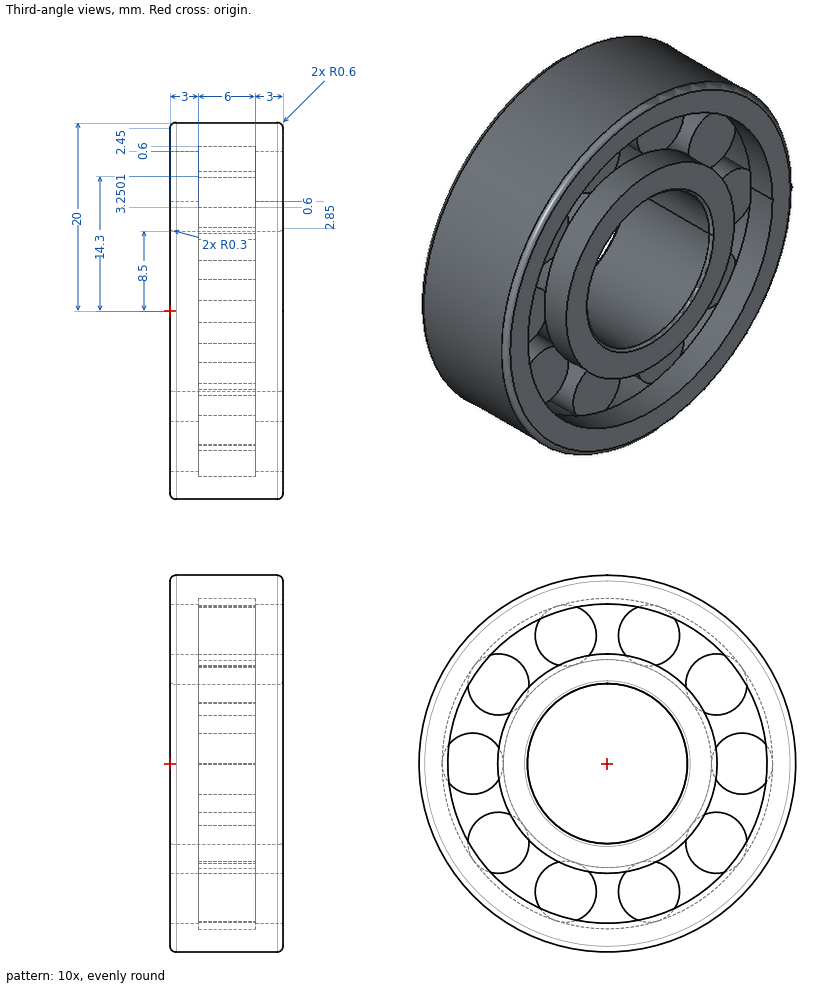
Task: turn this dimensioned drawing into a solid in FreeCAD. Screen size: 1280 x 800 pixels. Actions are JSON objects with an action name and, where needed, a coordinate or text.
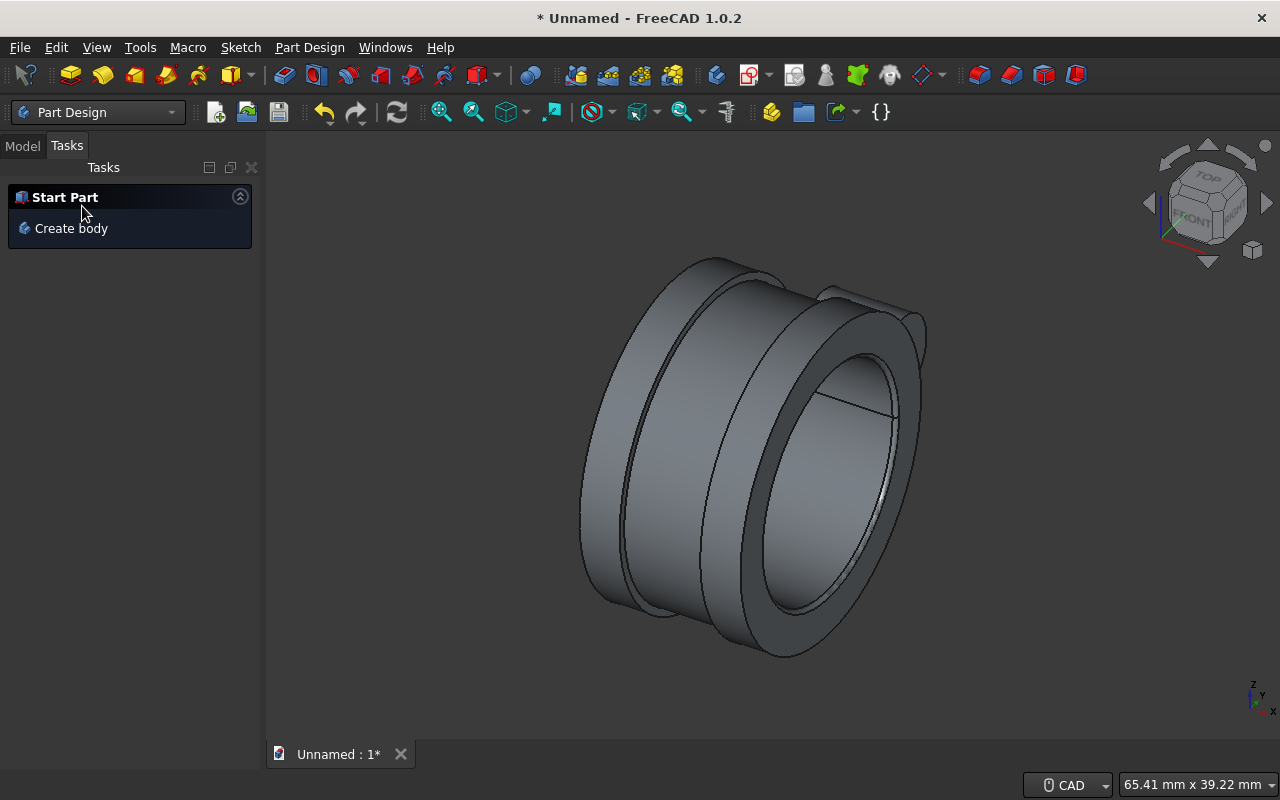
{"action": "left_click", "coordinate": [750, 76]}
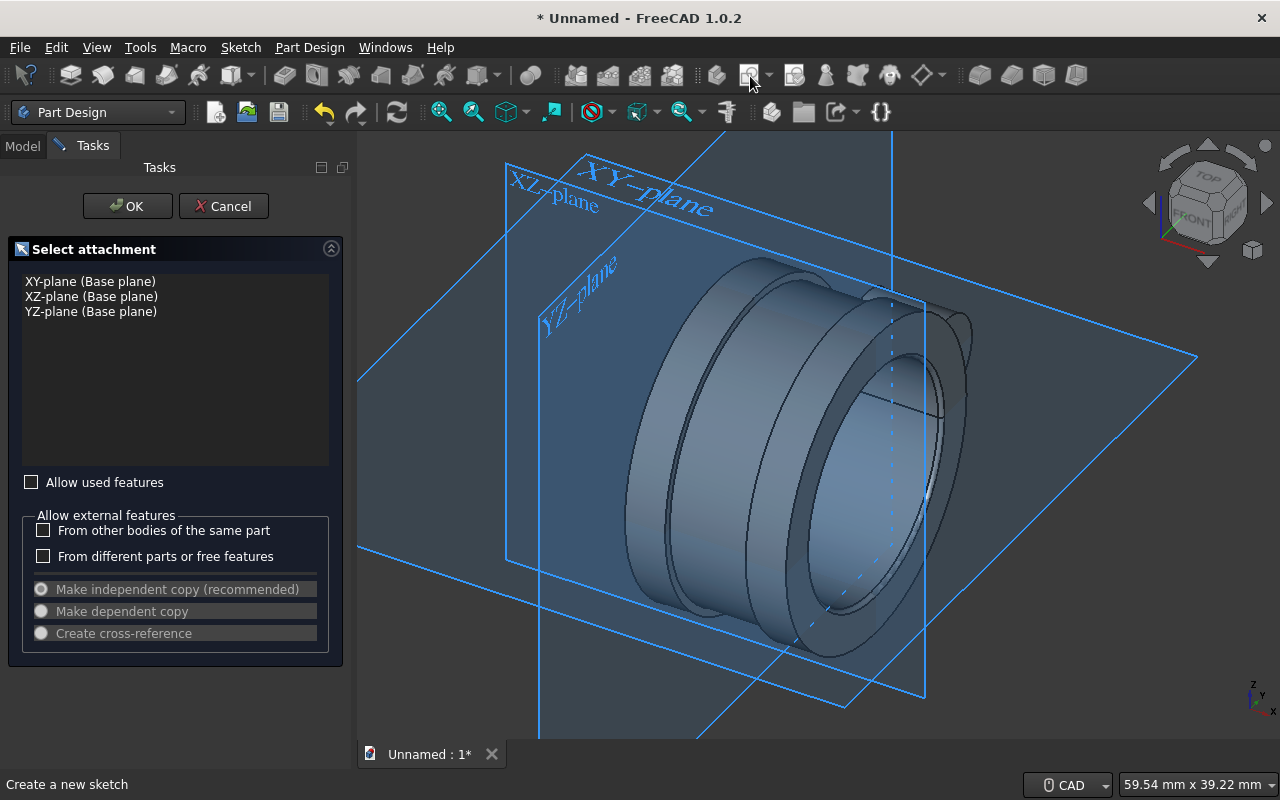
{"action": "left_click", "coordinate": [82, 282]}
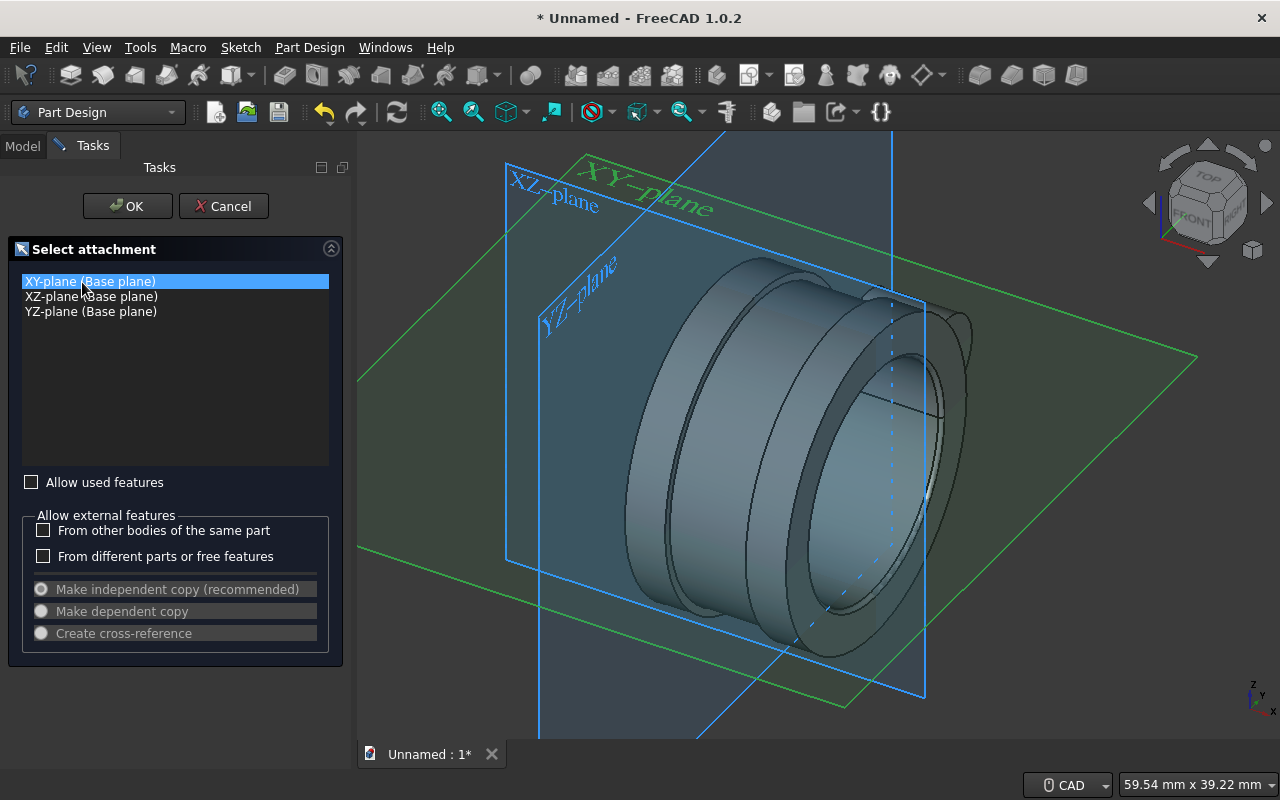
{"action": "left_click", "coordinate": [128, 206]}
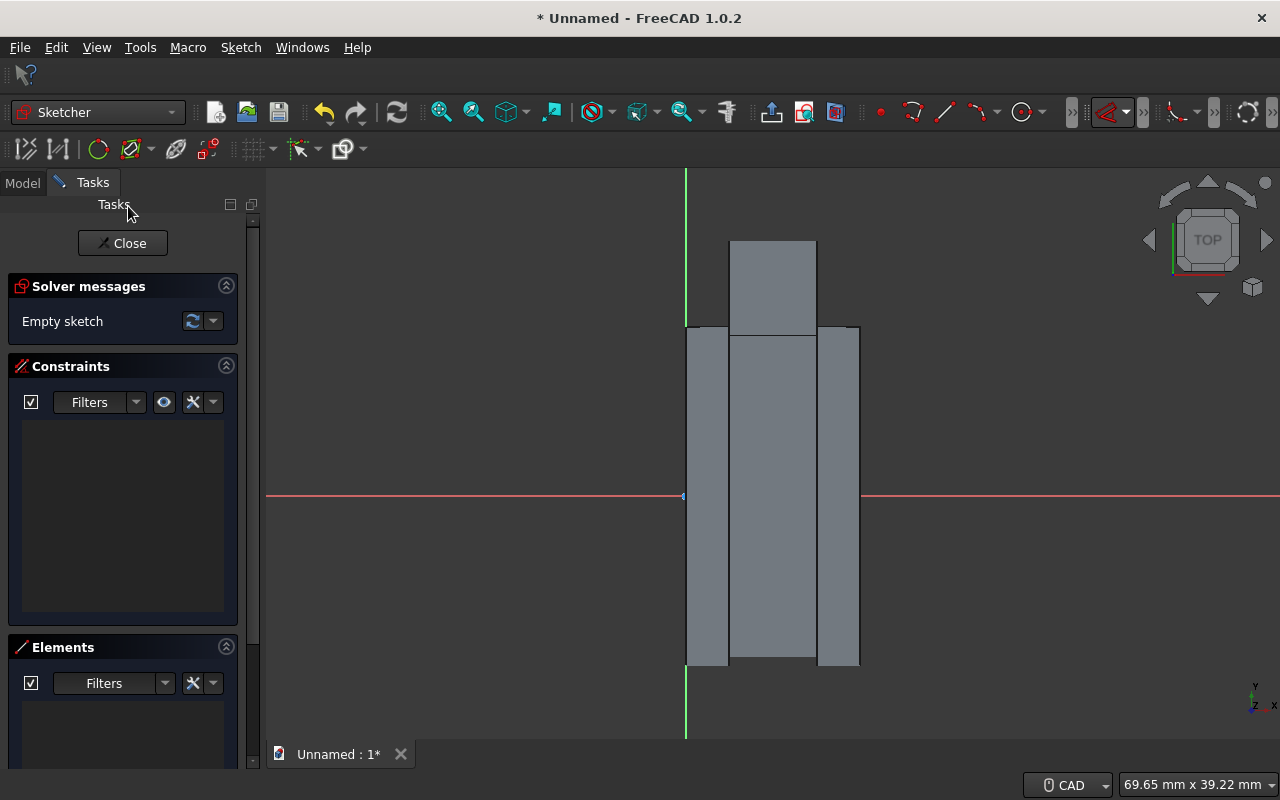
{"action": "left_click", "coordinate": [836, 112]}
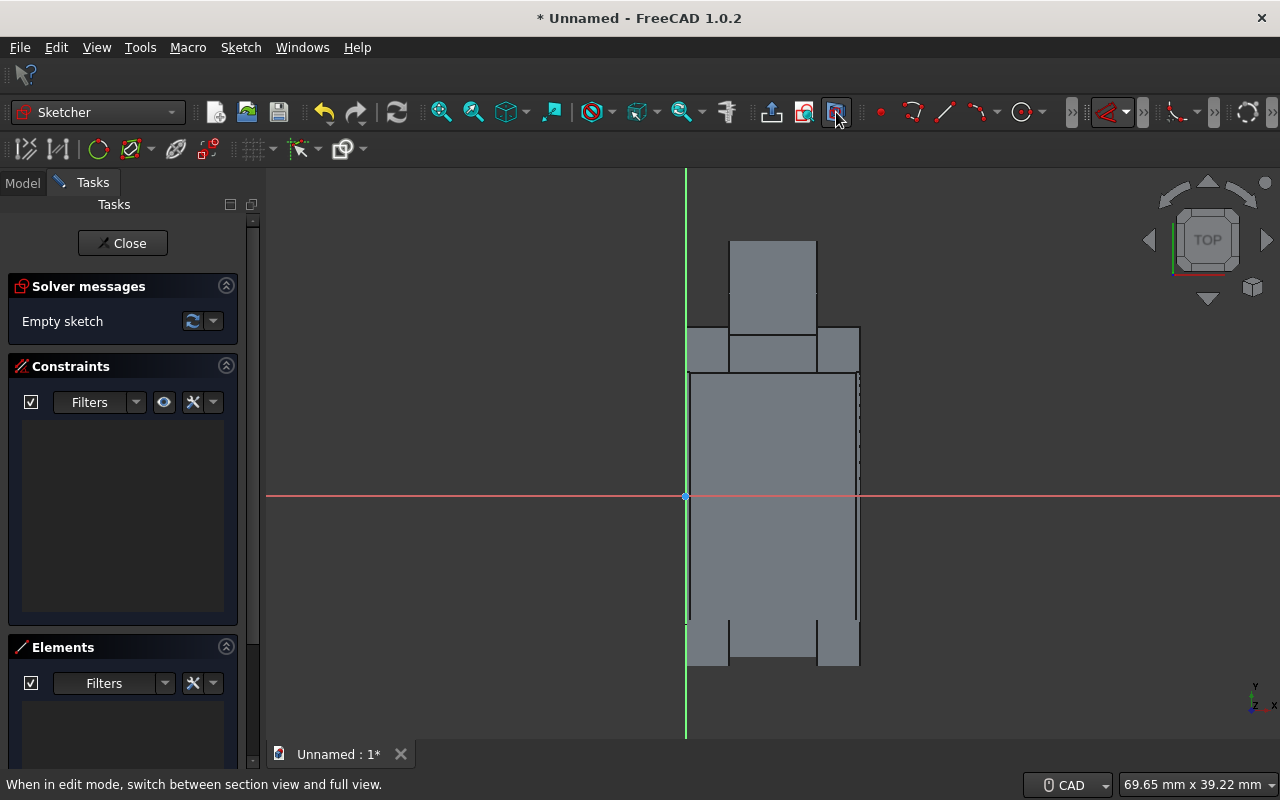
{"action": "scroll", "coordinate": [395, 711], "scroll_direction": "down", "scroll_amount": 1}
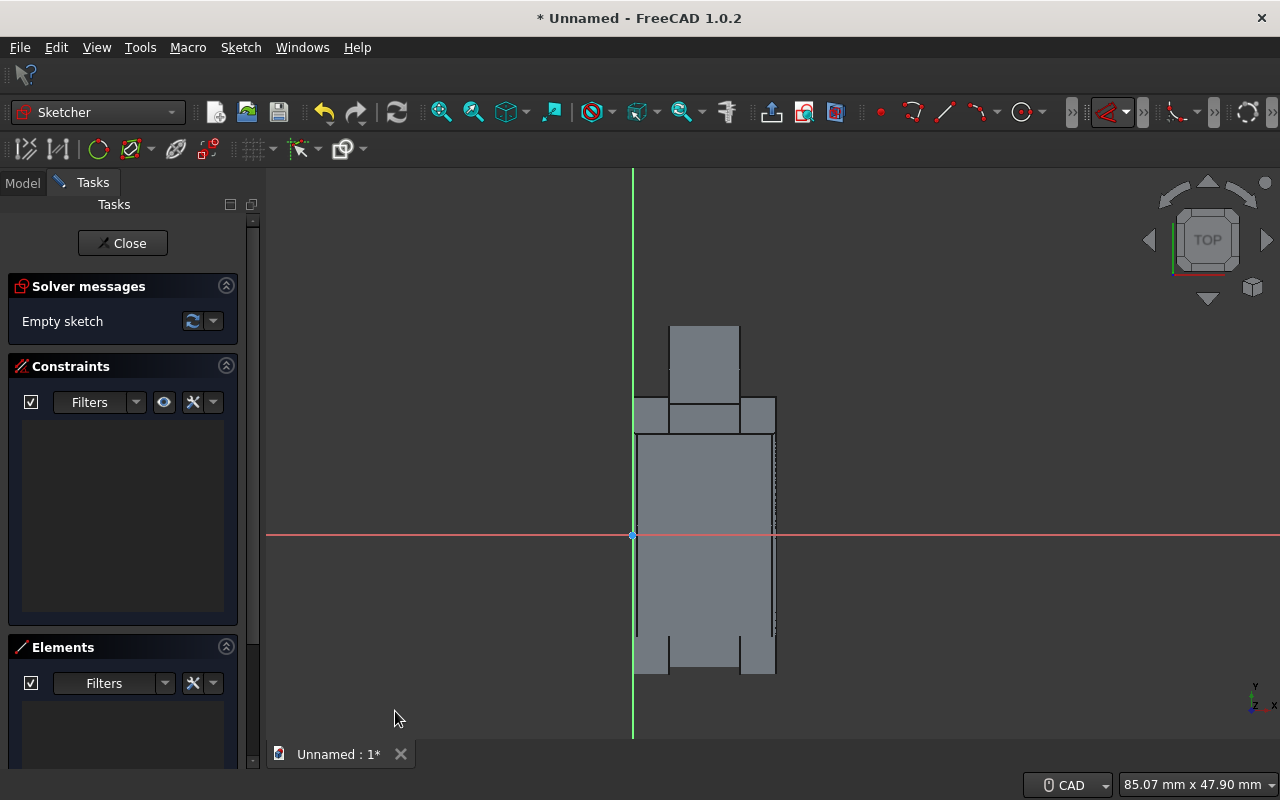
{"action": "scroll", "coordinate": [705, 340], "scroll_direction": "up", "scroll_amount": 2}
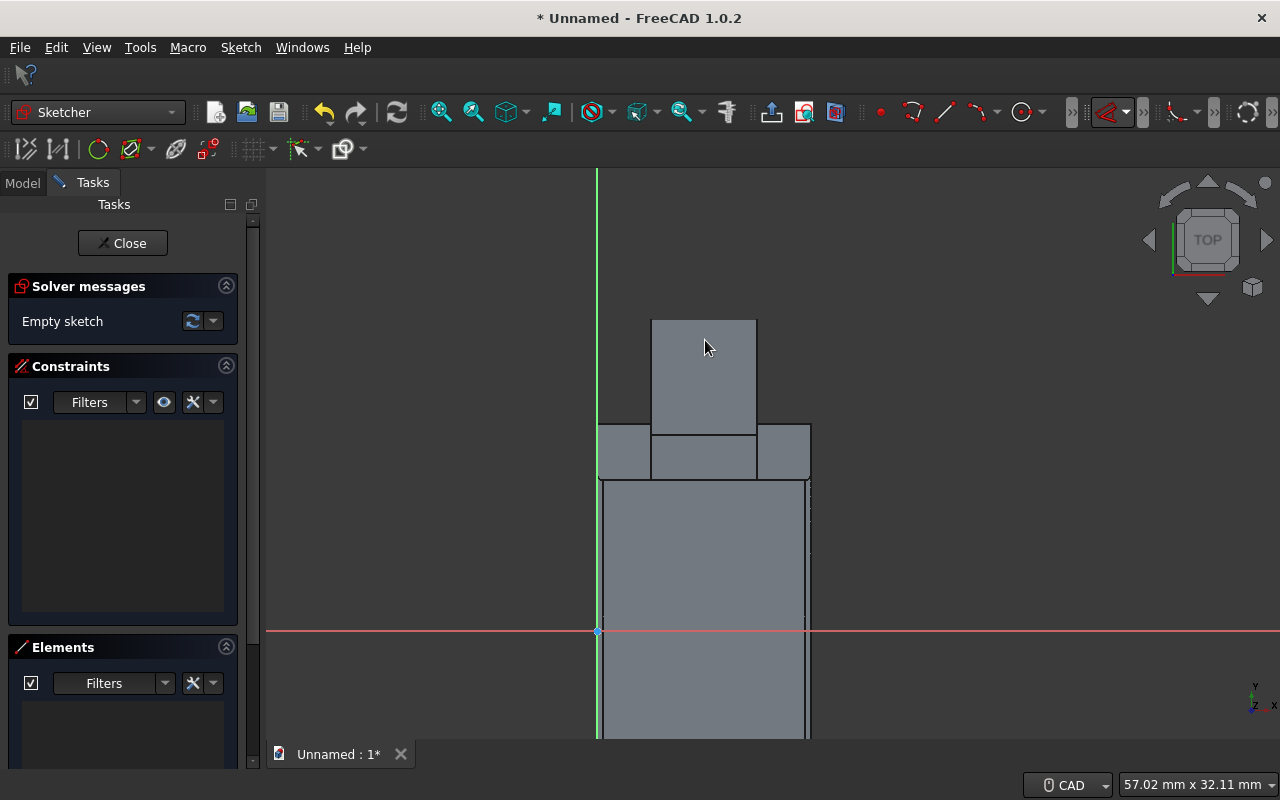
{"action": "left_click", "coordinate": [946, 112]}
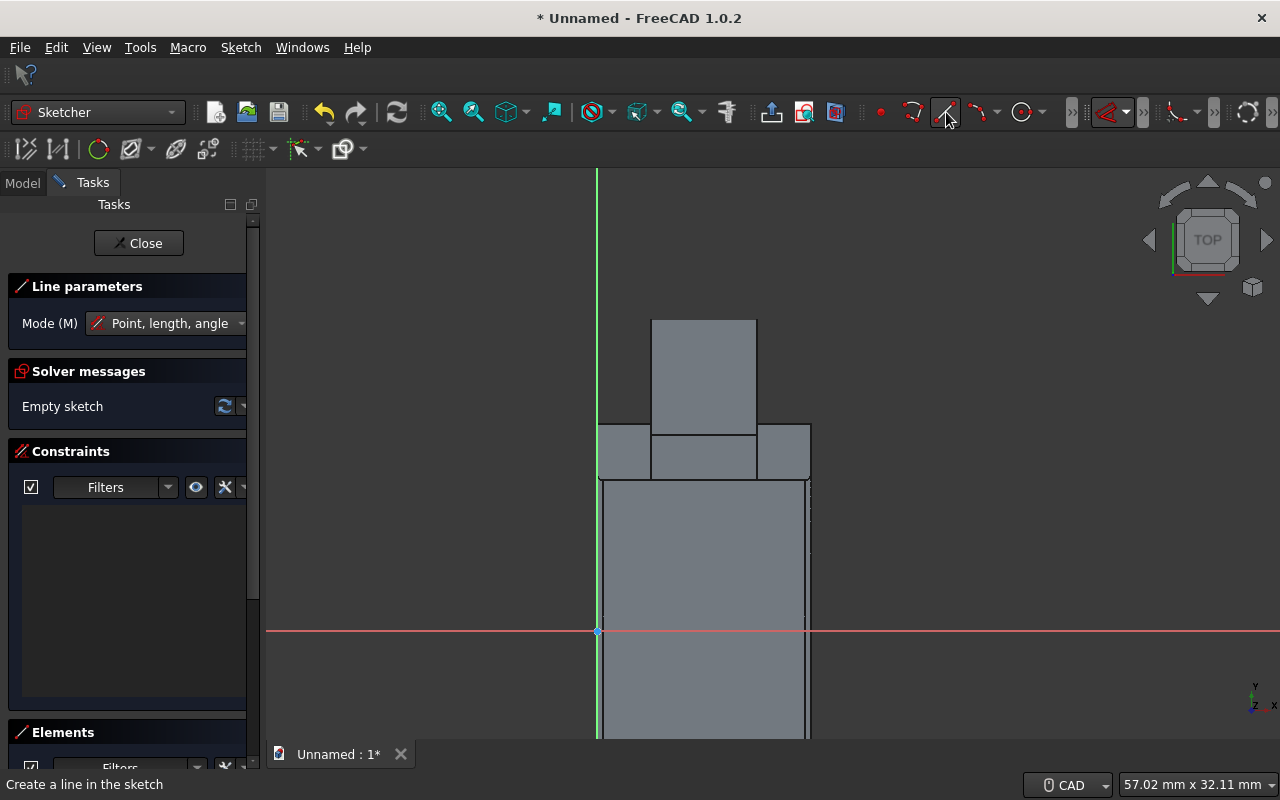
{"action": "left_click", "coordinate": [800, 276]}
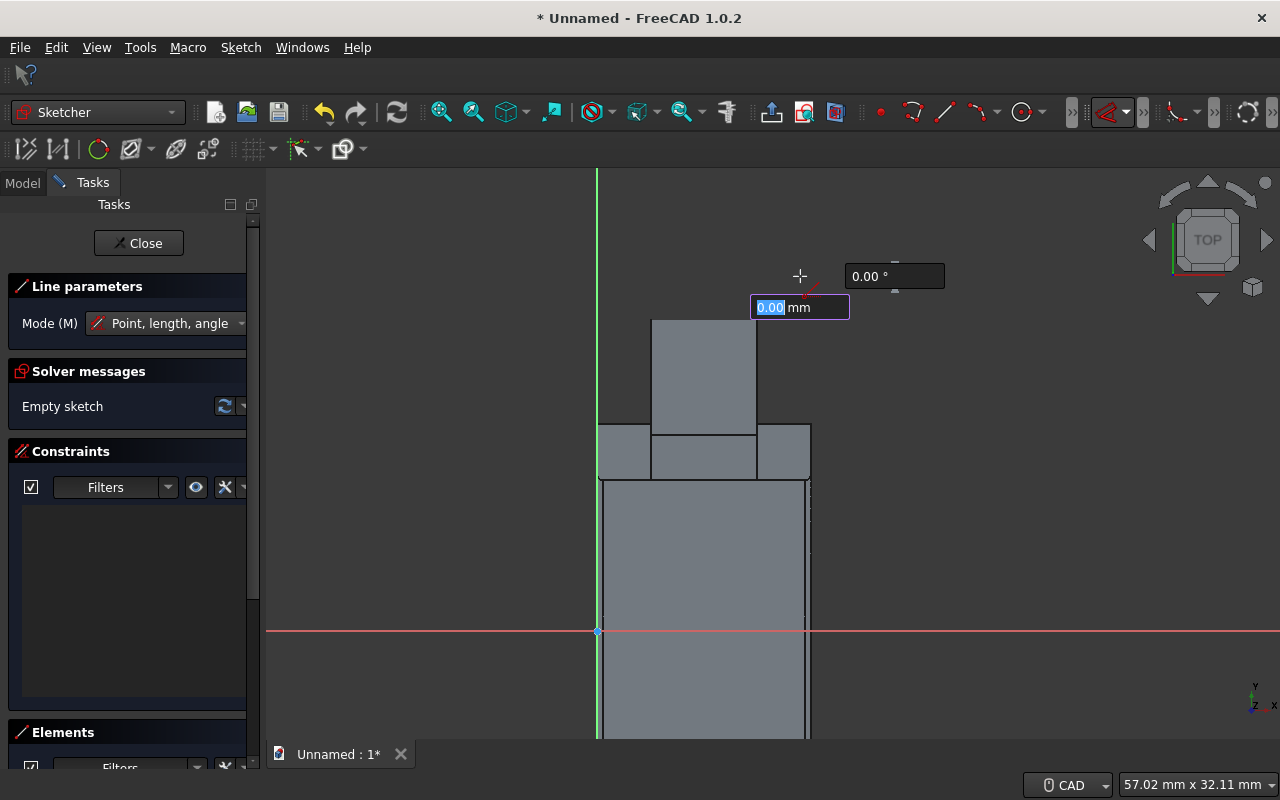
{"action": "scroll", "coordinate": [608, 276], "scroll_direction": "up", "scroll_amount": 2}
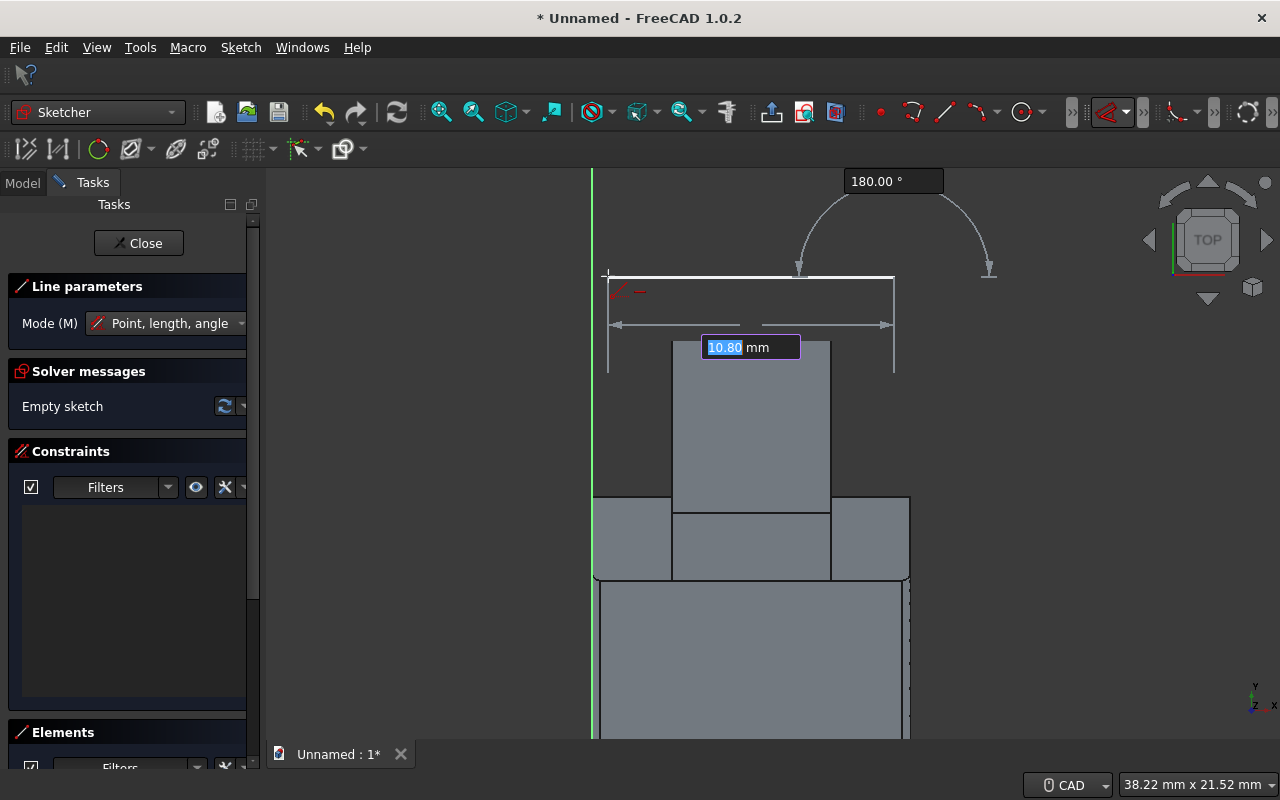
{"action": "left_click", "coordinate": [608, 276]}